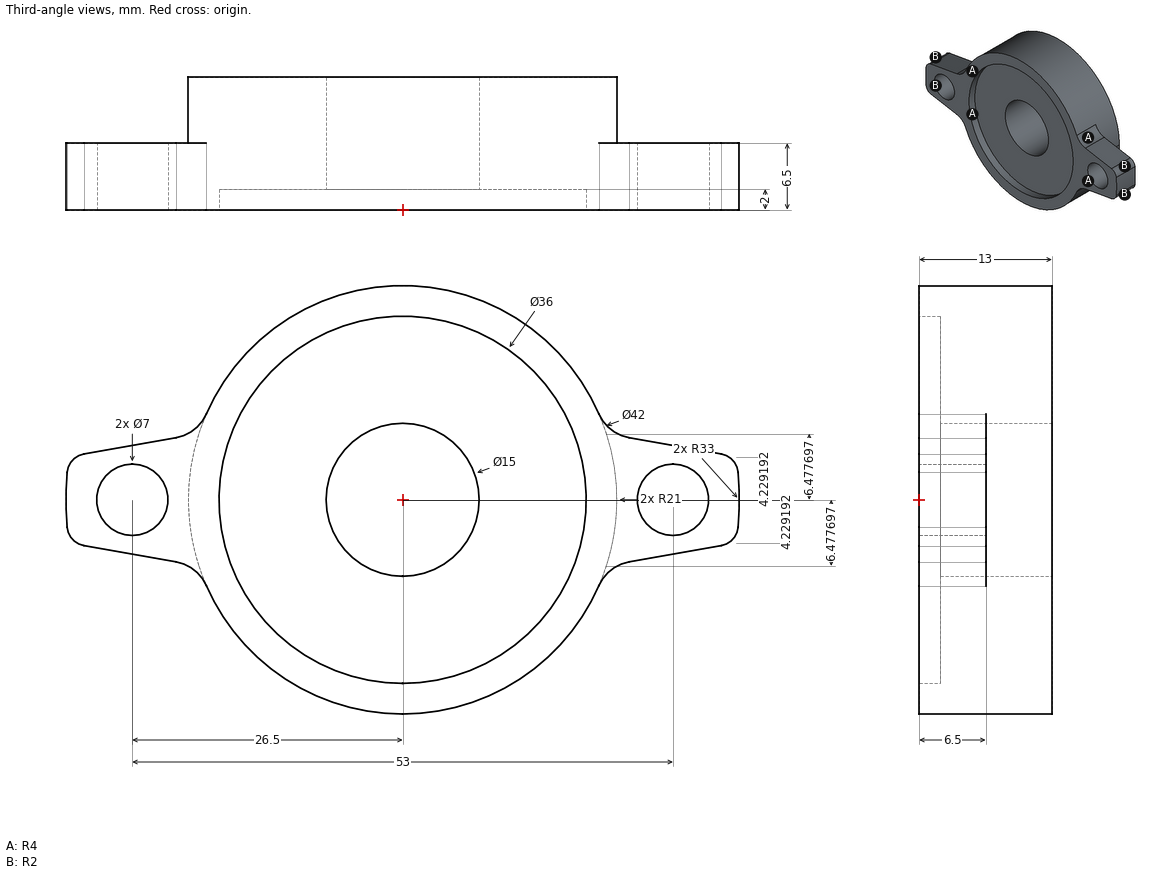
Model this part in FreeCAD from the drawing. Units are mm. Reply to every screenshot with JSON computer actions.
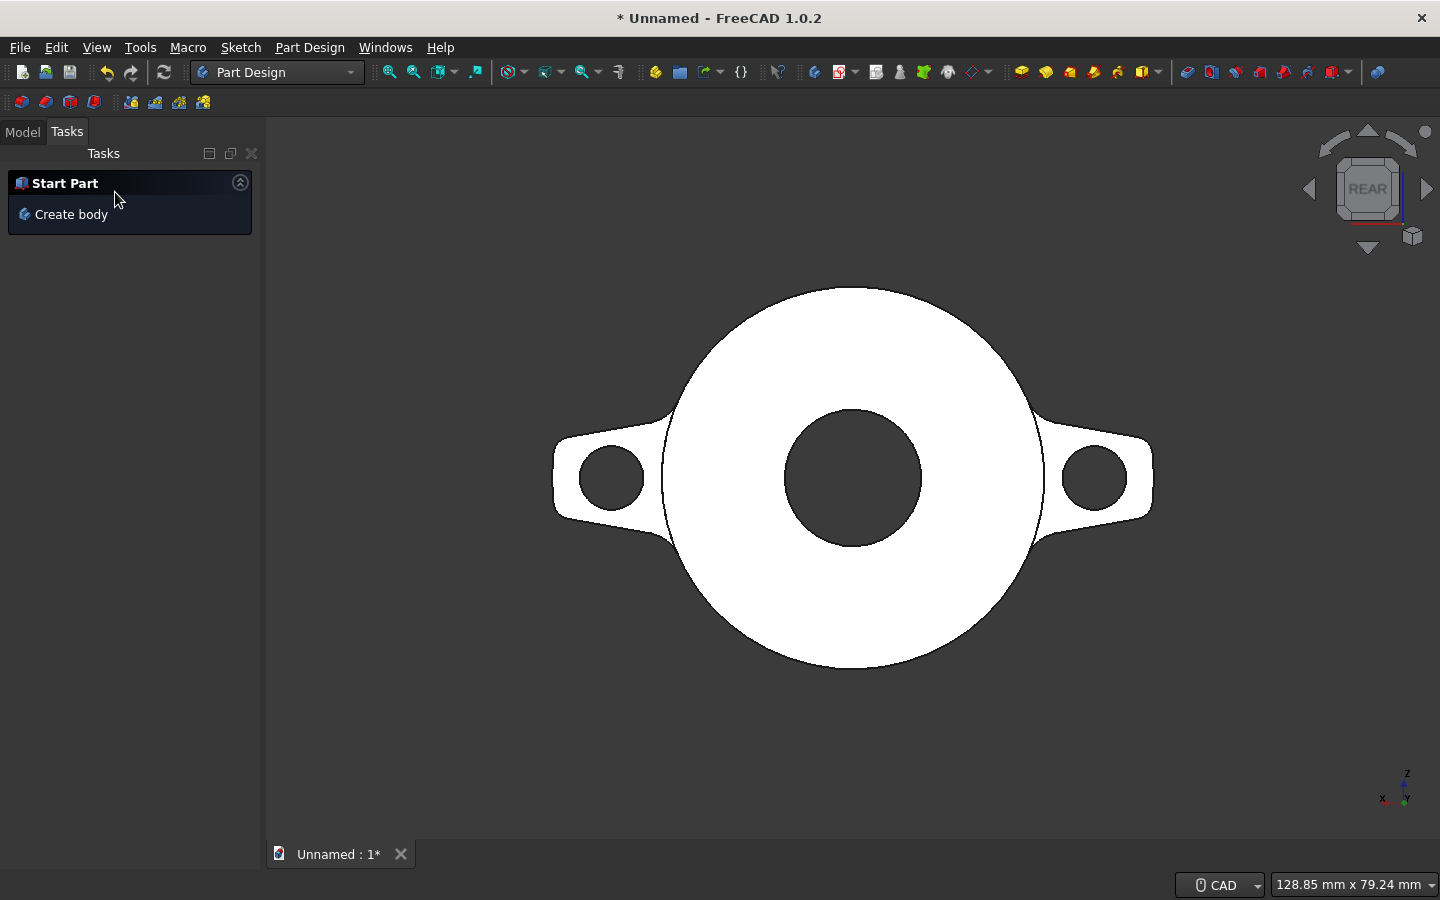
{"action": "key", "text": "0"}